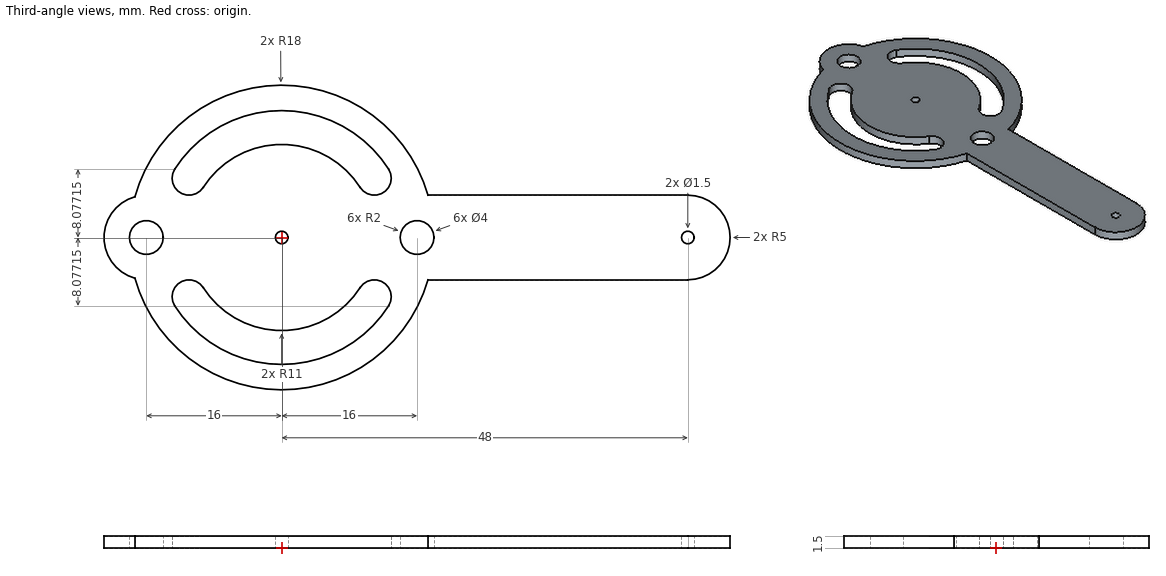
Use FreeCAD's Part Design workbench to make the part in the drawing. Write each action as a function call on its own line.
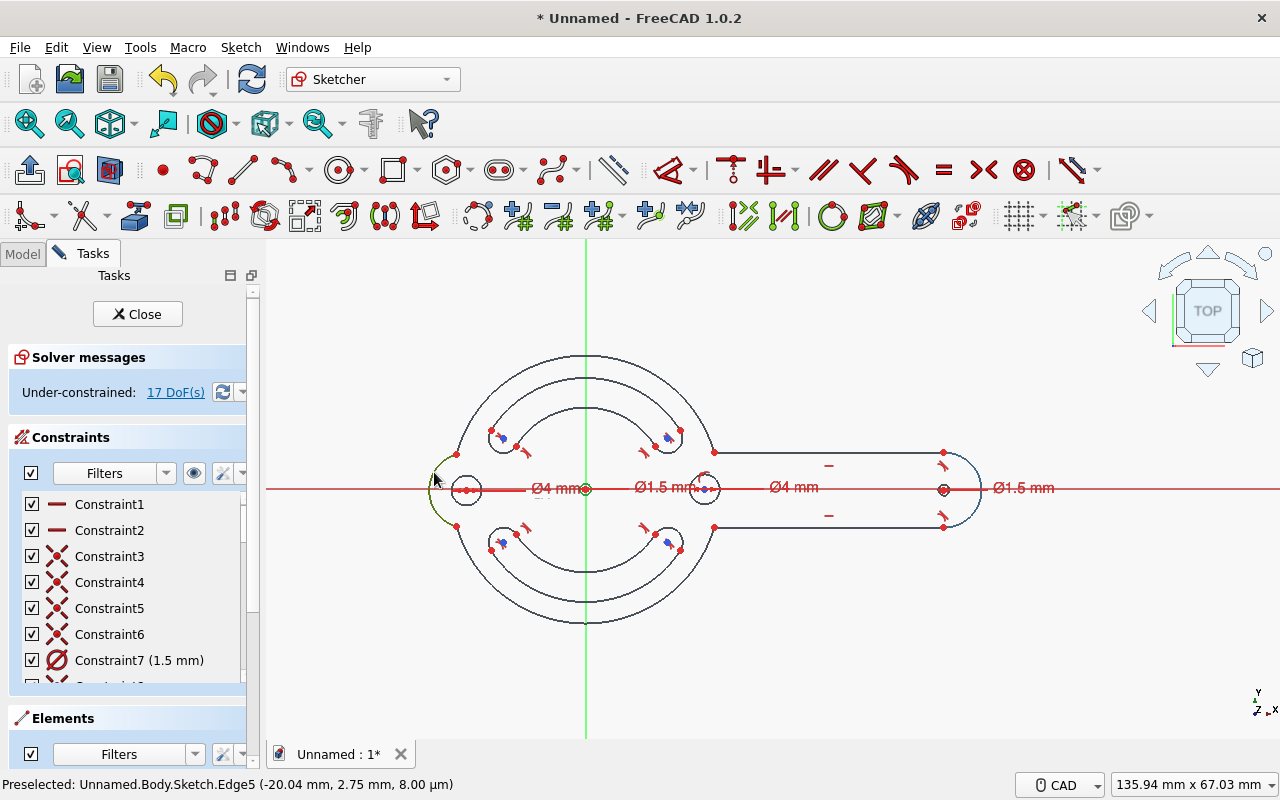
click(944, 170)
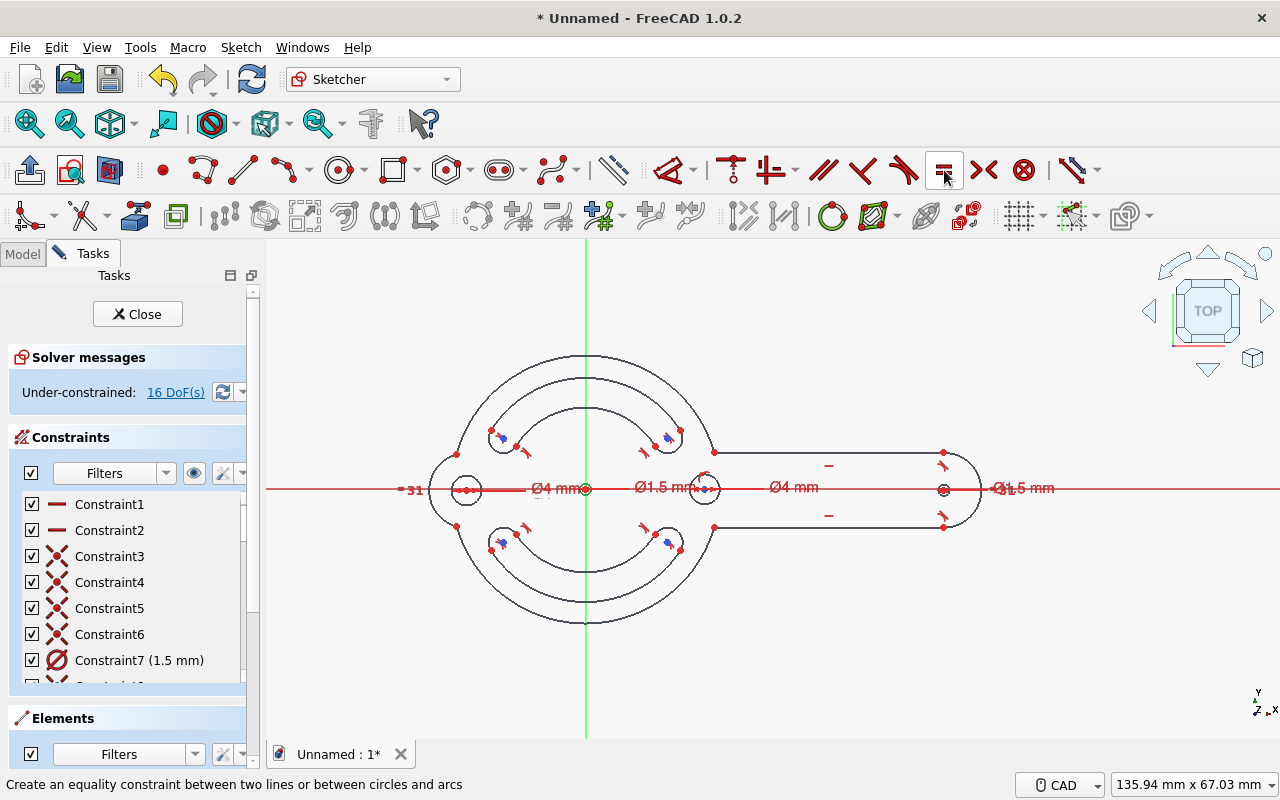
click(651, 373)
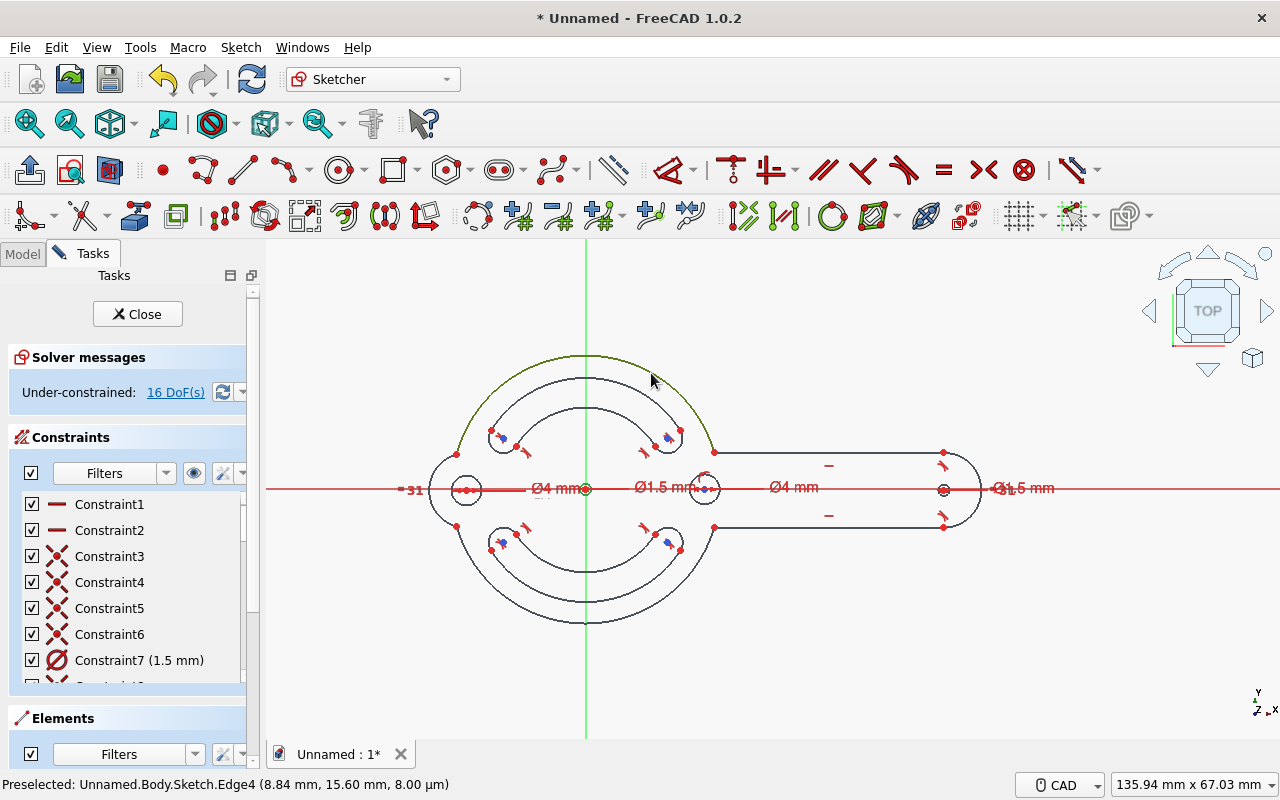
click(519, 606)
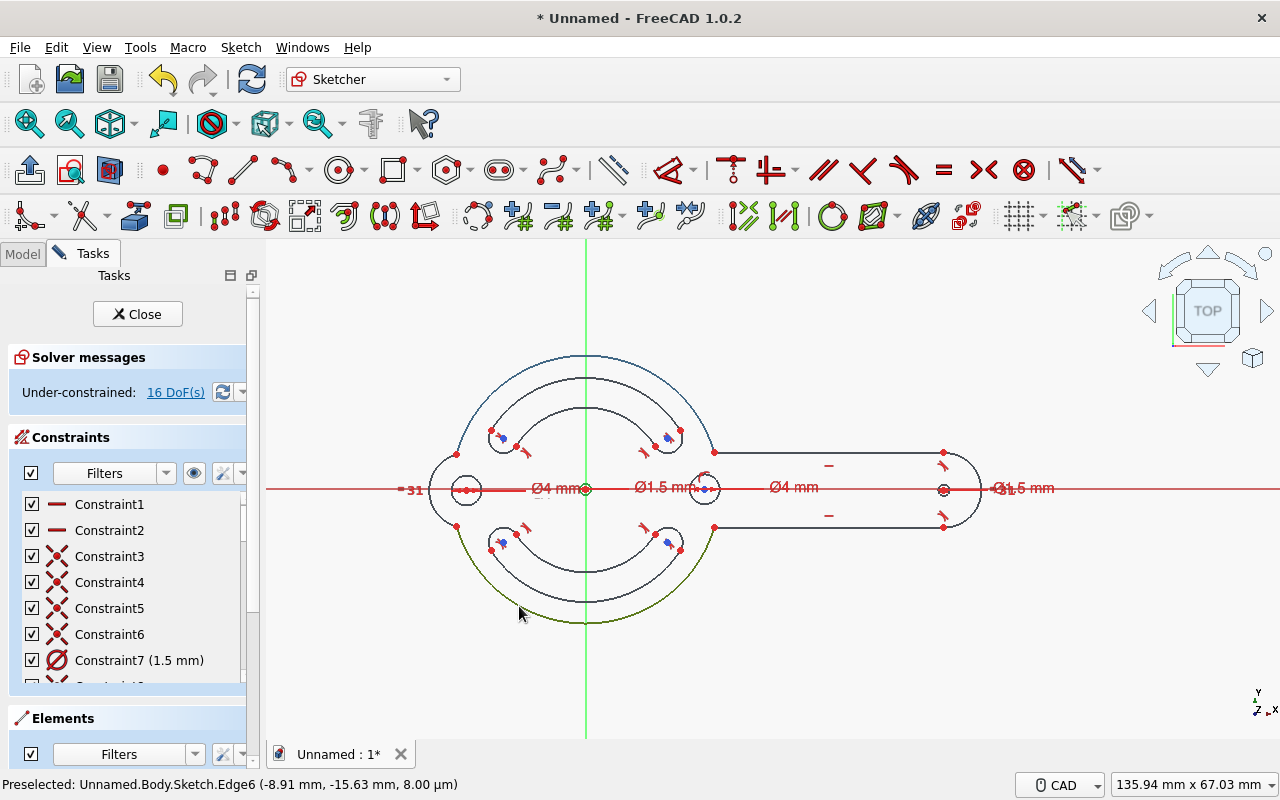
click(944, 170)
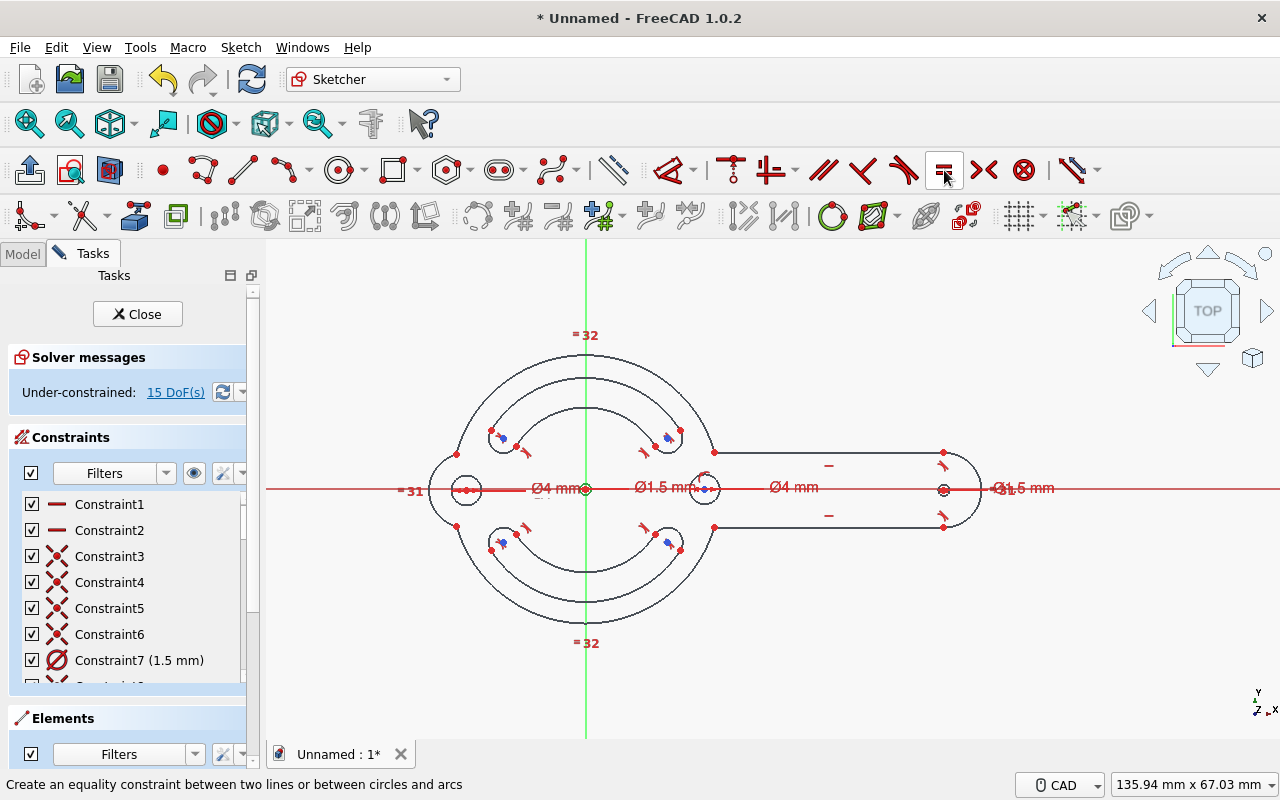
click(553, 566)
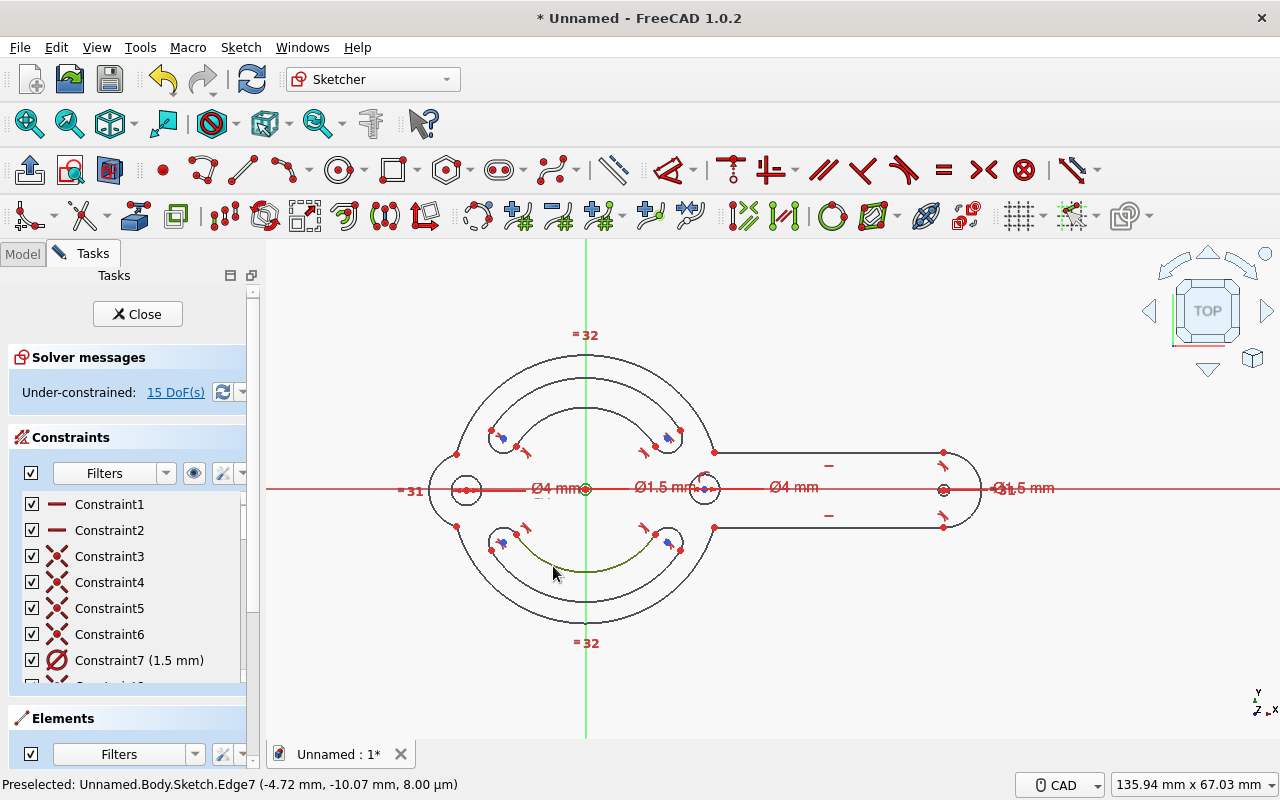
click(618, 414)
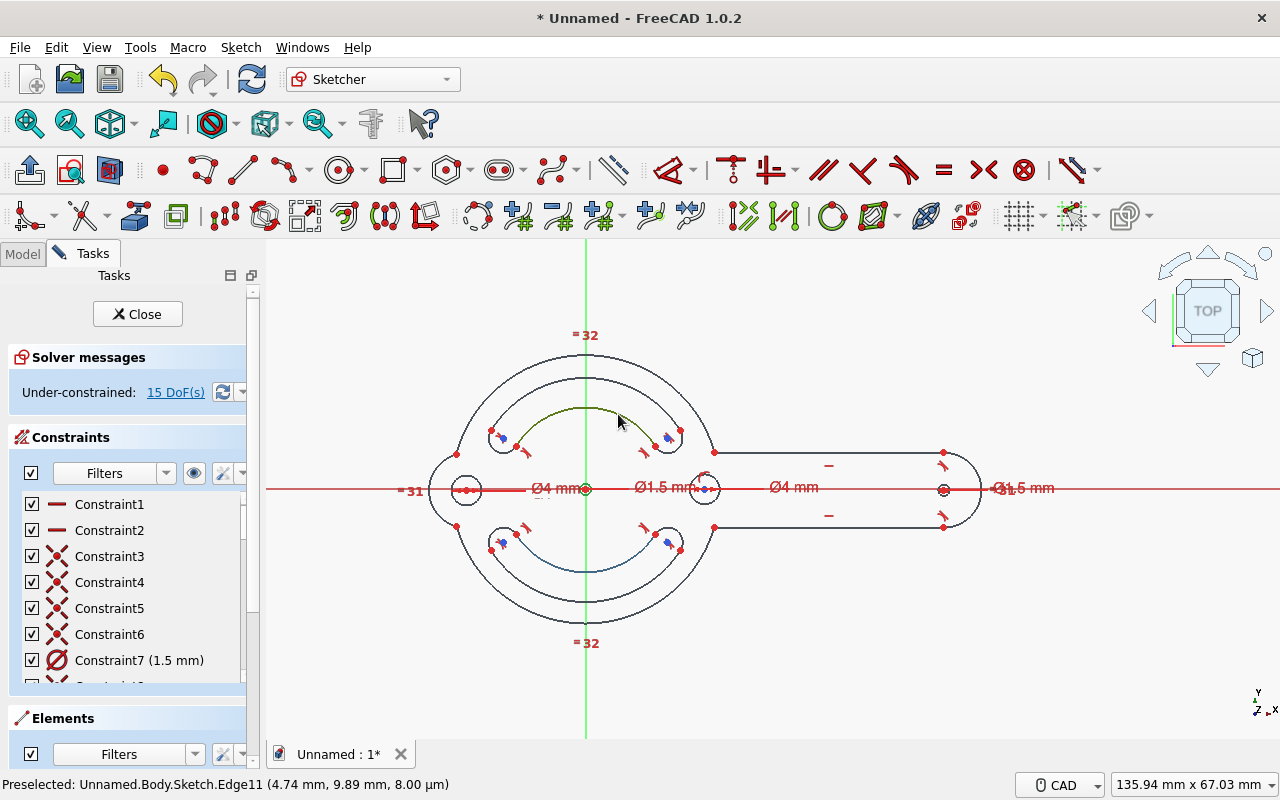
click(944, 170)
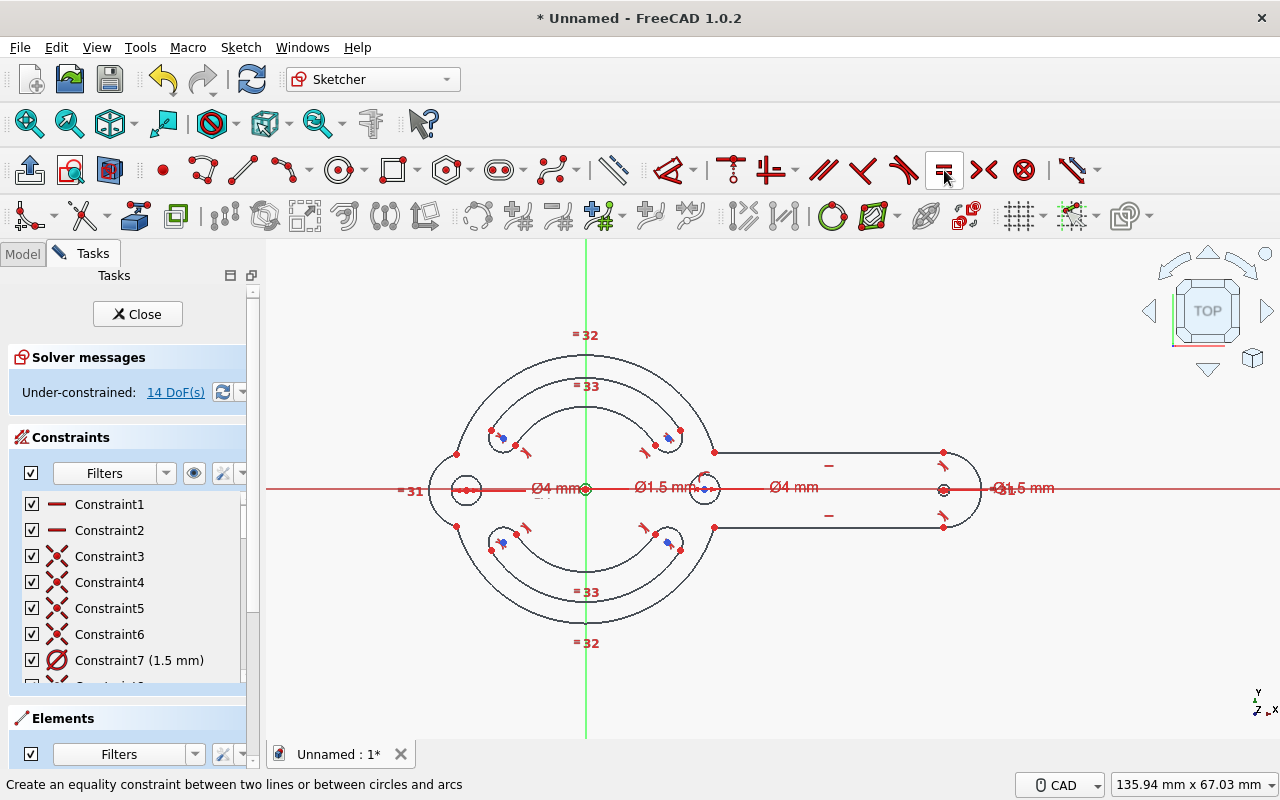
click(682, 537)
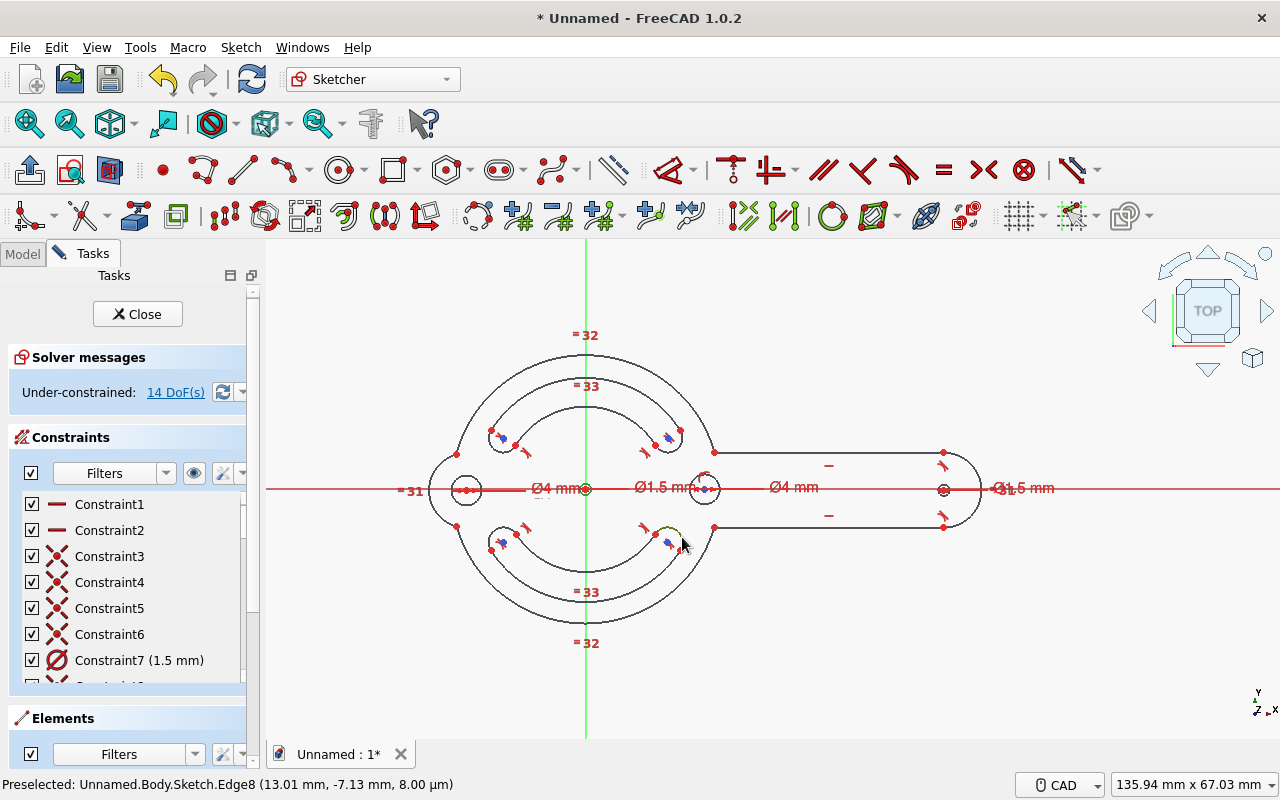
click(490, 444)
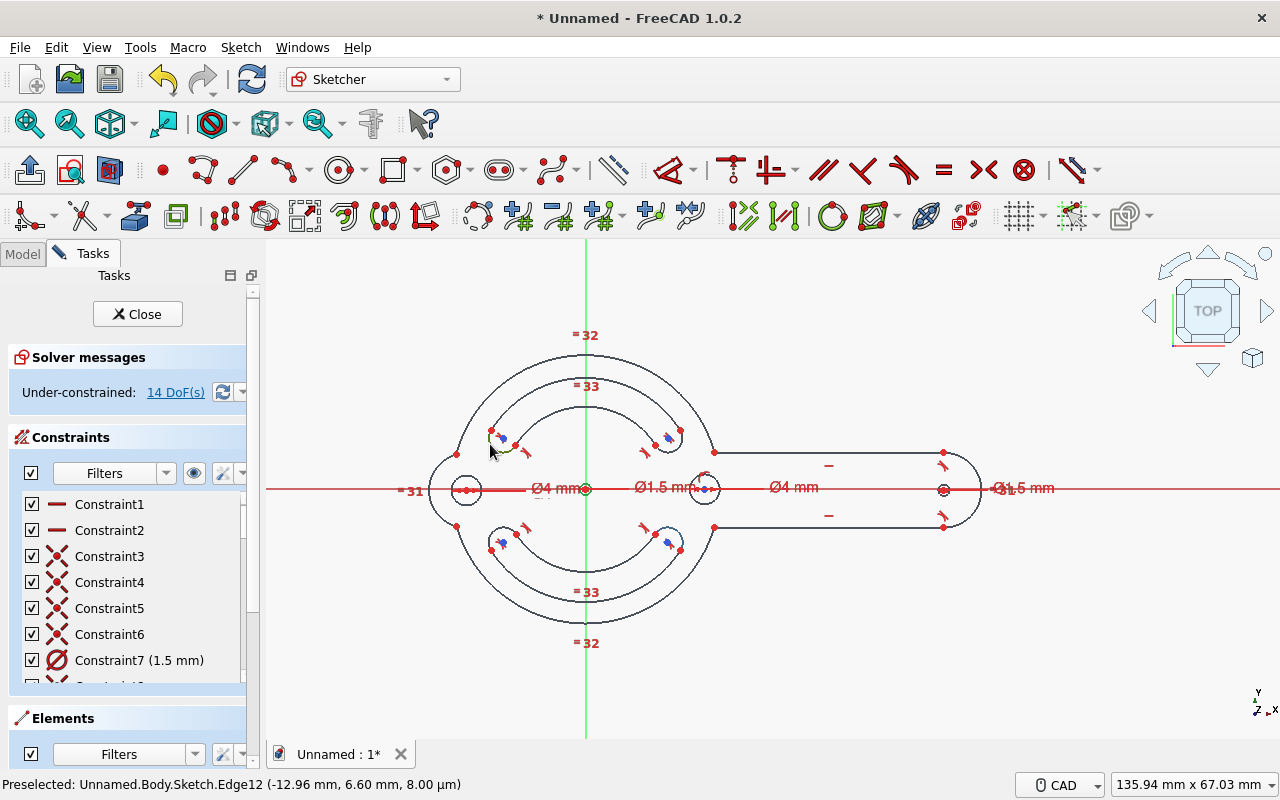
click(944, 170)